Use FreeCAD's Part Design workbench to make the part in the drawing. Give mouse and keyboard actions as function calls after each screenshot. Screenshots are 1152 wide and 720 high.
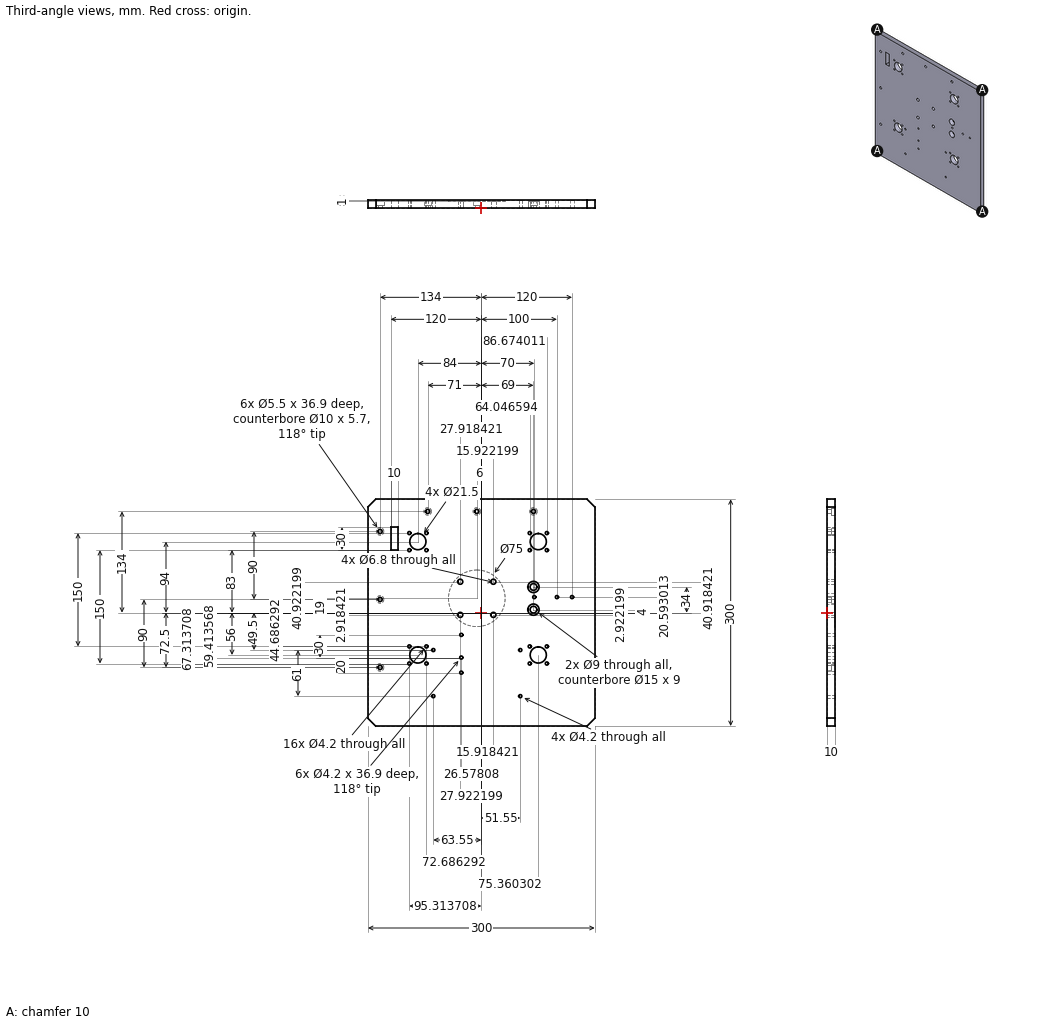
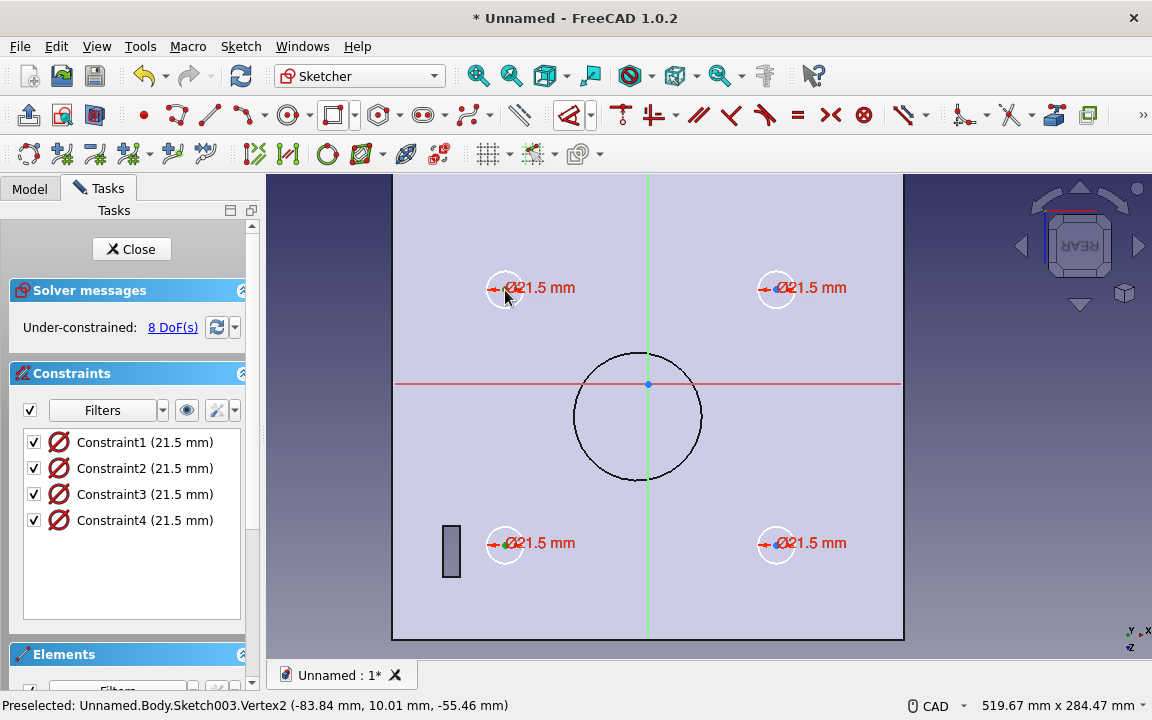
click(676, 116)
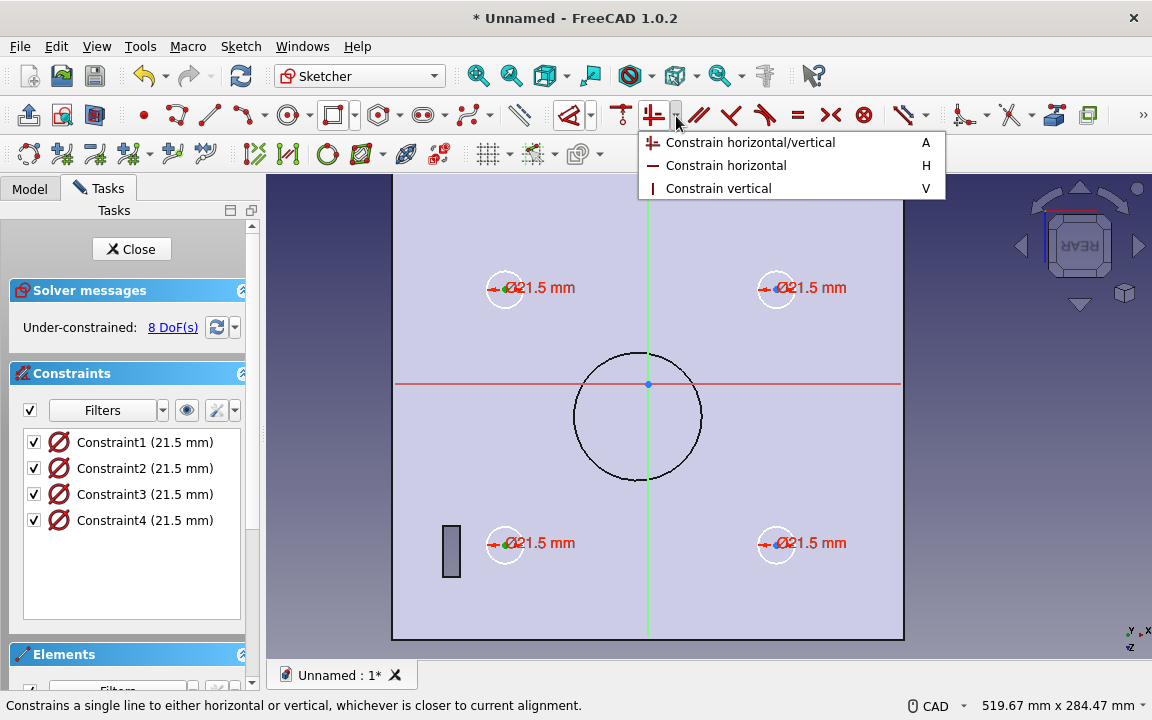
click(792, 188)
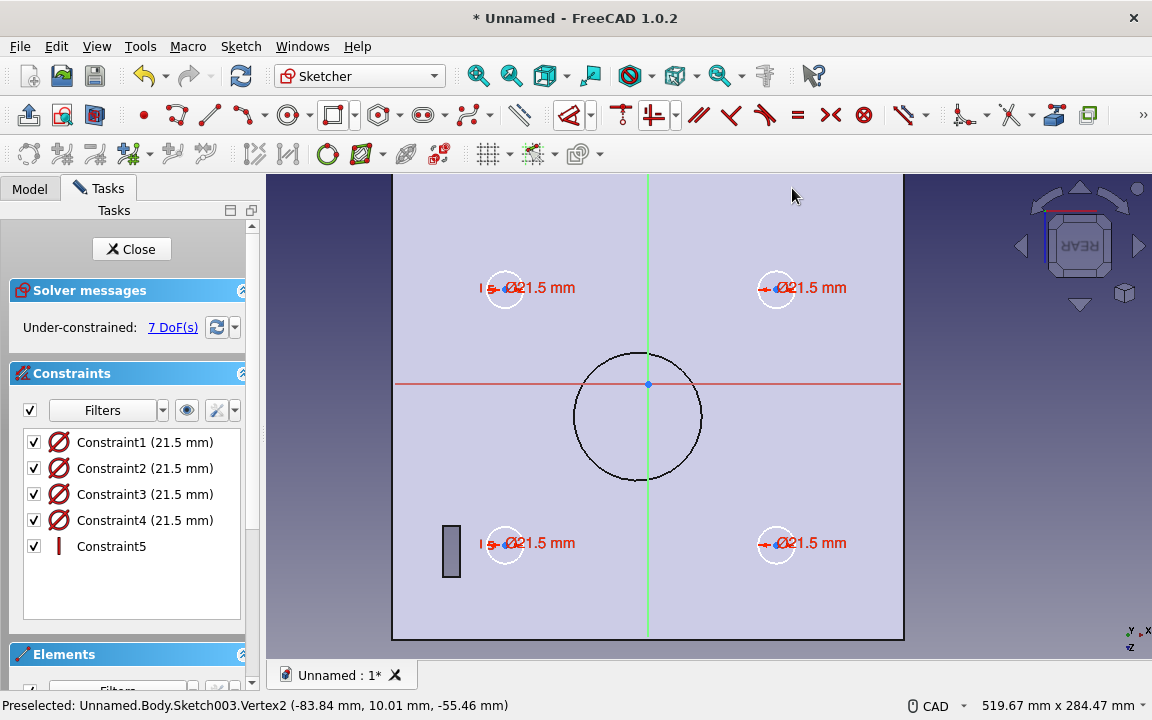
click(505, 290)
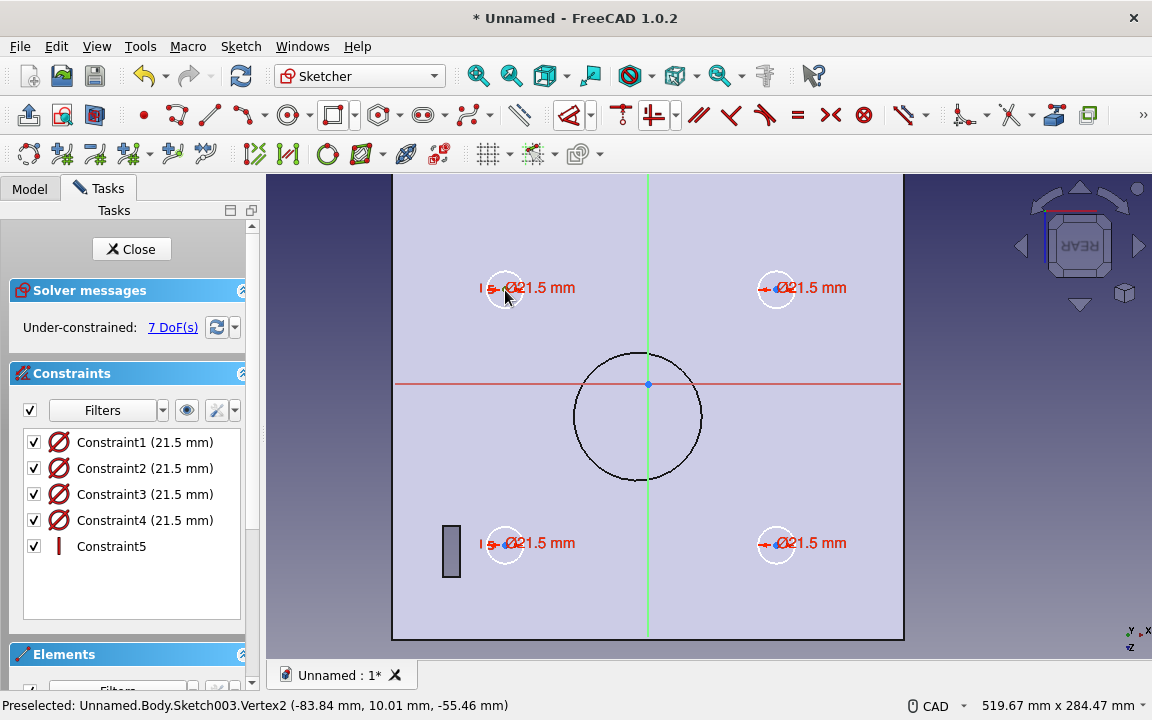
click(777, 290)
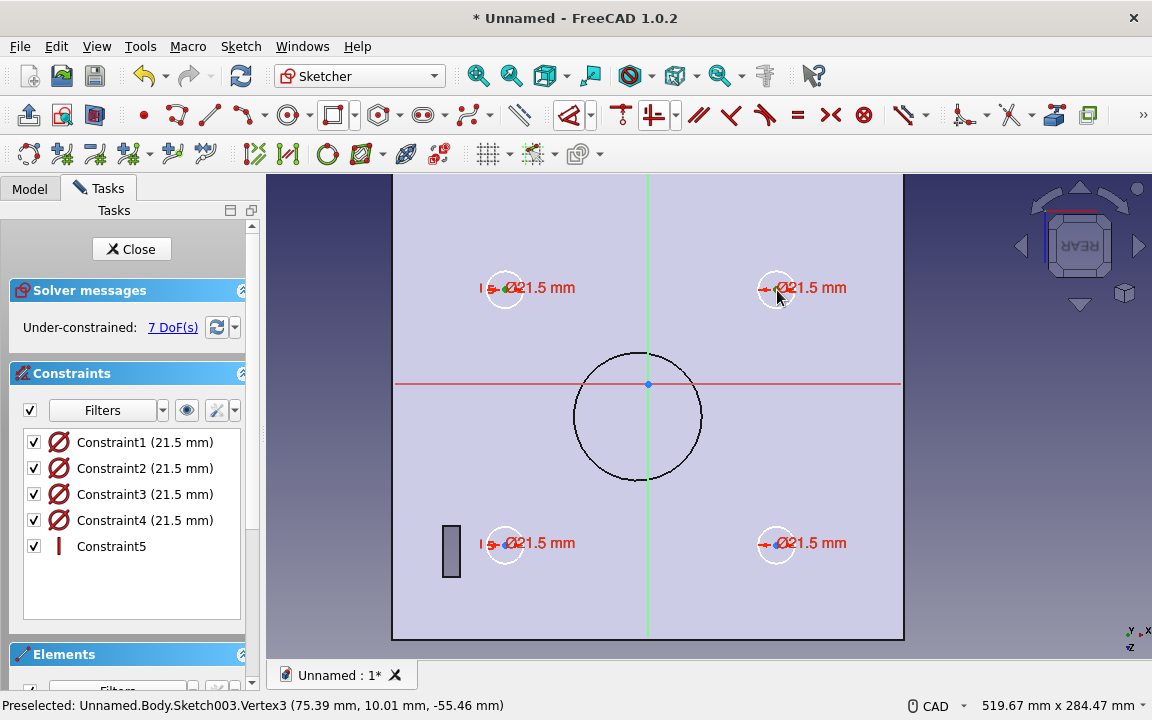
key(h)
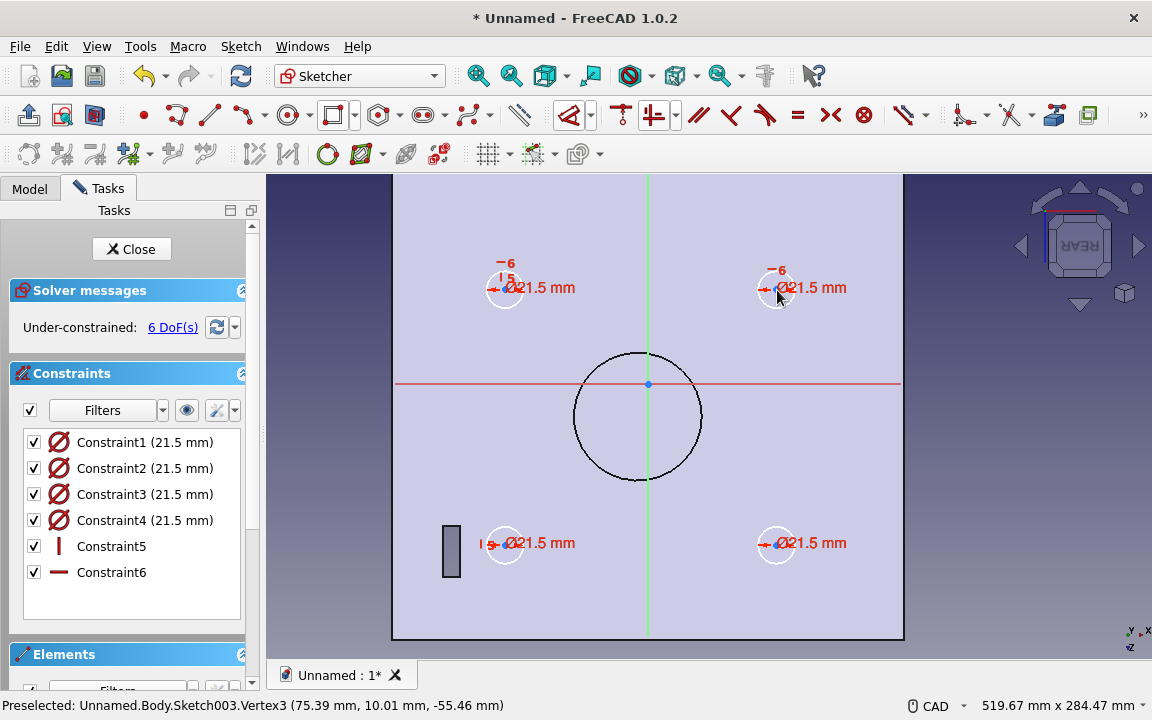
click(777, 290)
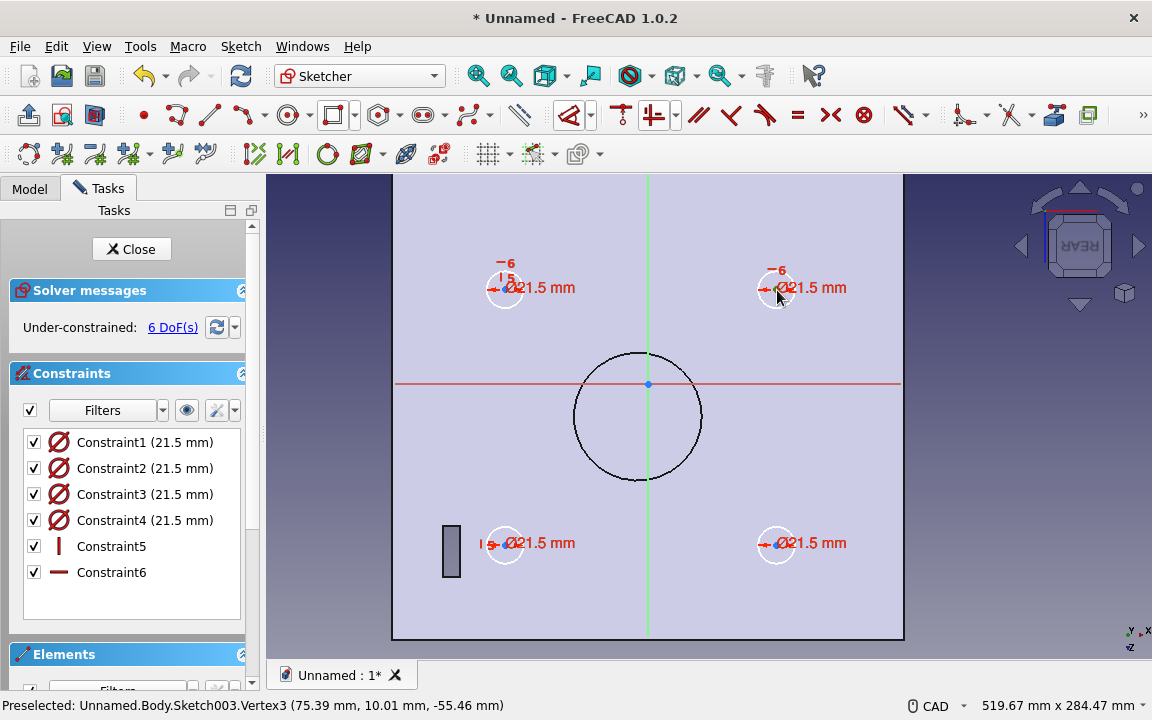
click(777, 545)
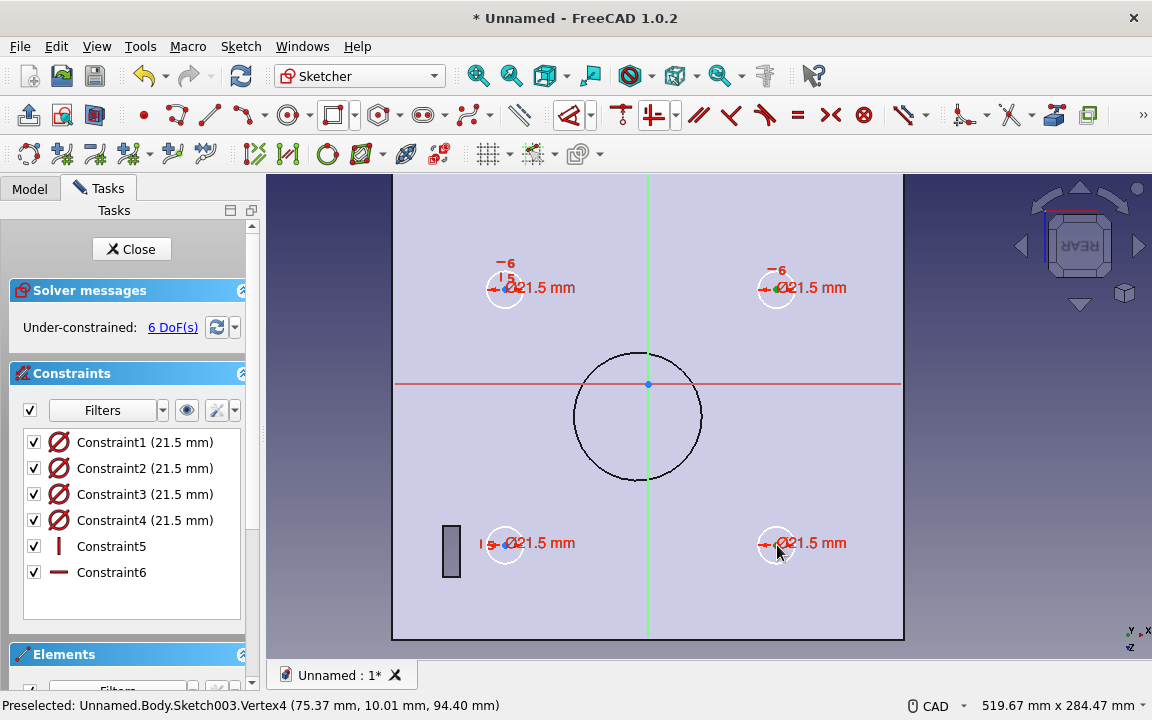
key(v)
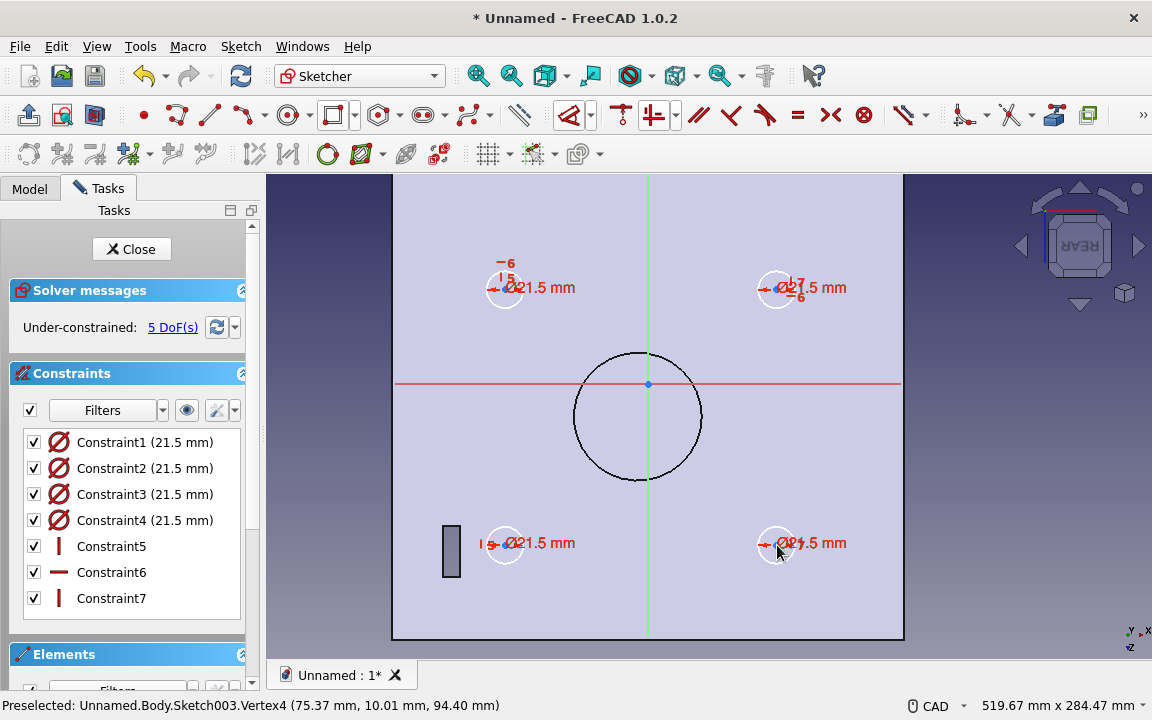
click(505, 545)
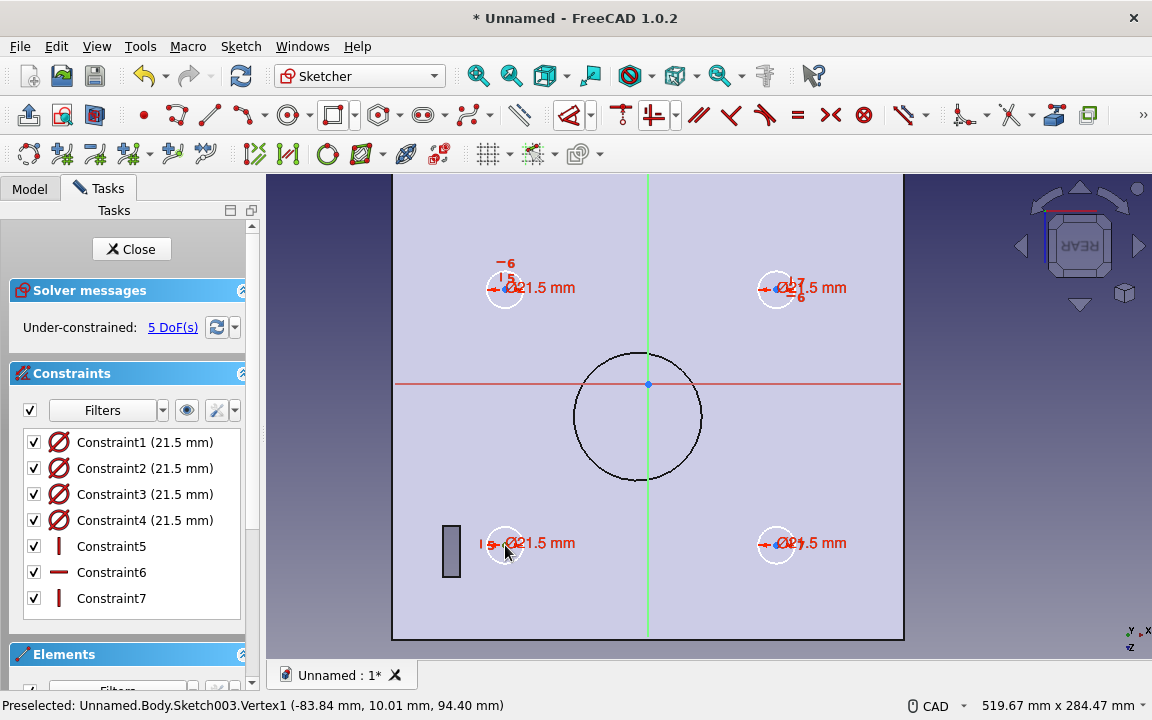
click(777, 545)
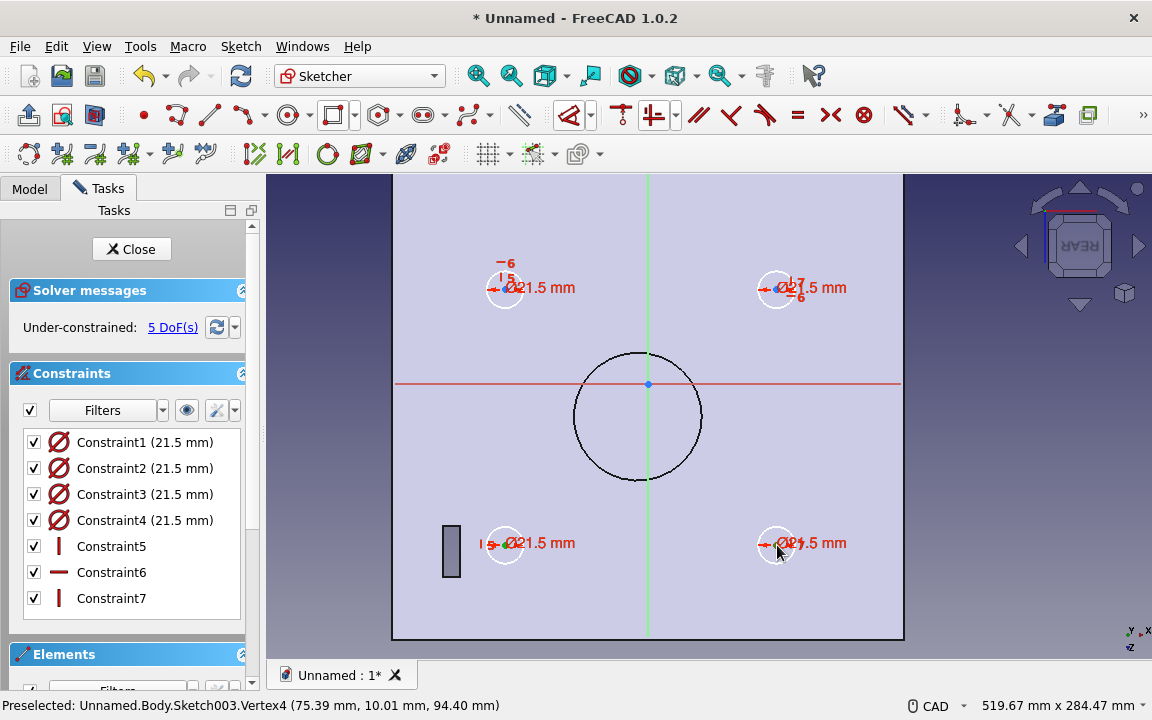
key(h)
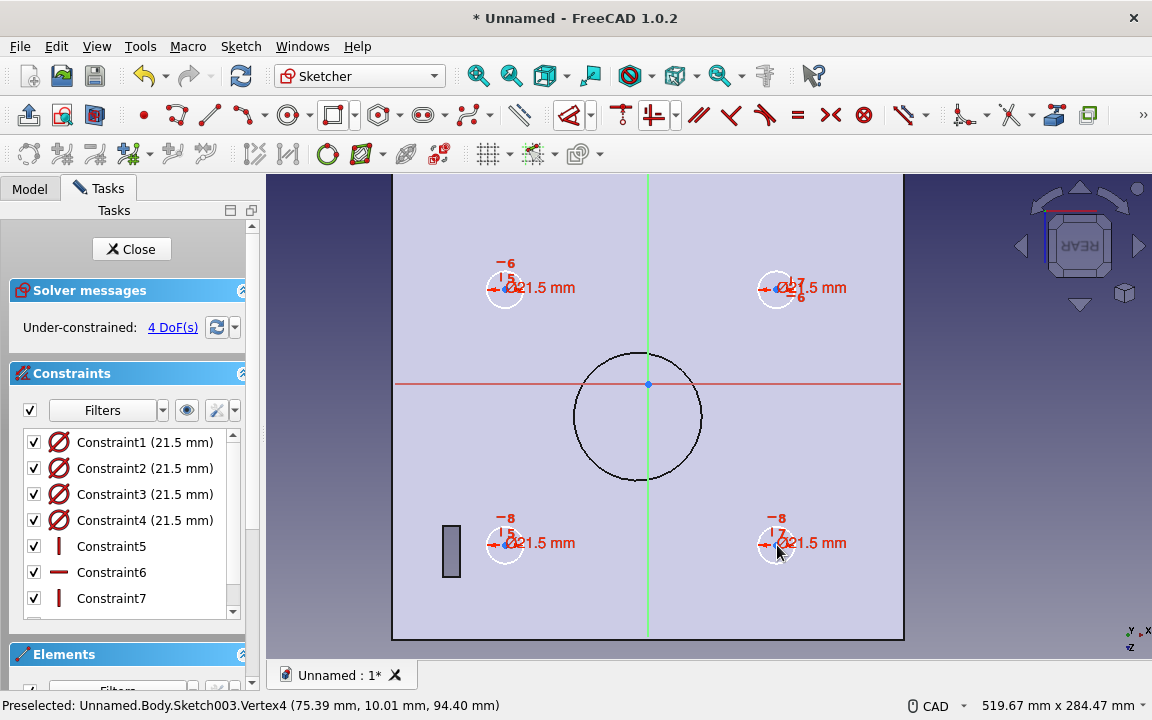
click(505, 545)